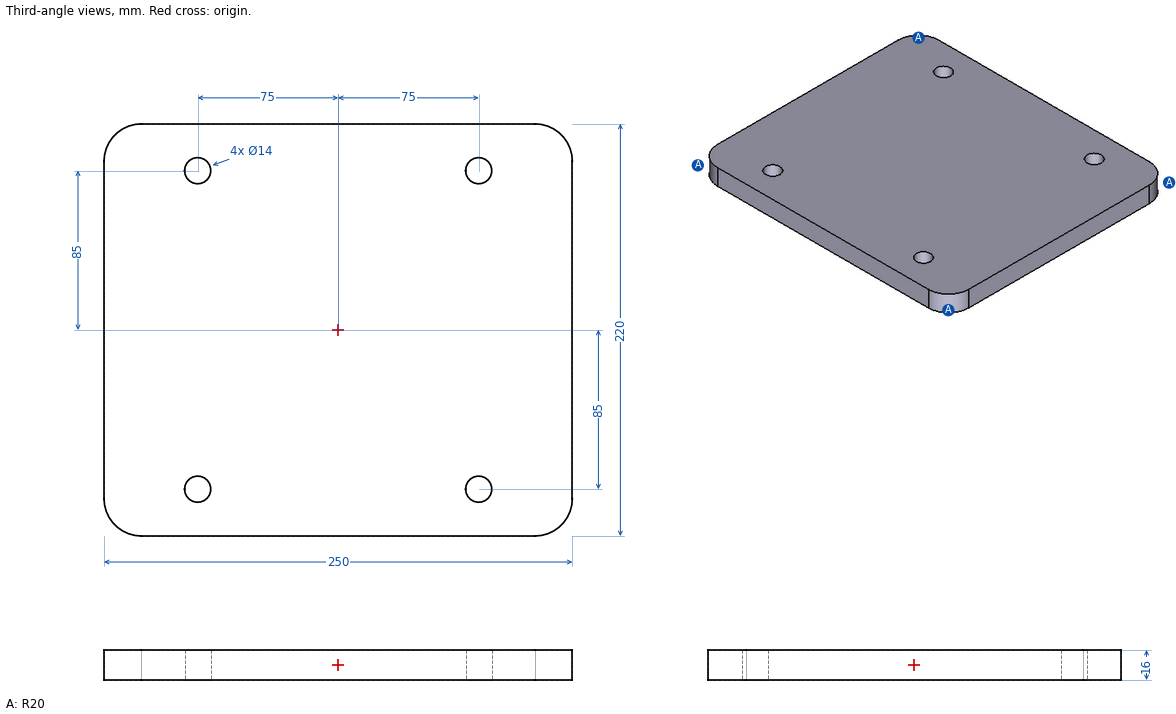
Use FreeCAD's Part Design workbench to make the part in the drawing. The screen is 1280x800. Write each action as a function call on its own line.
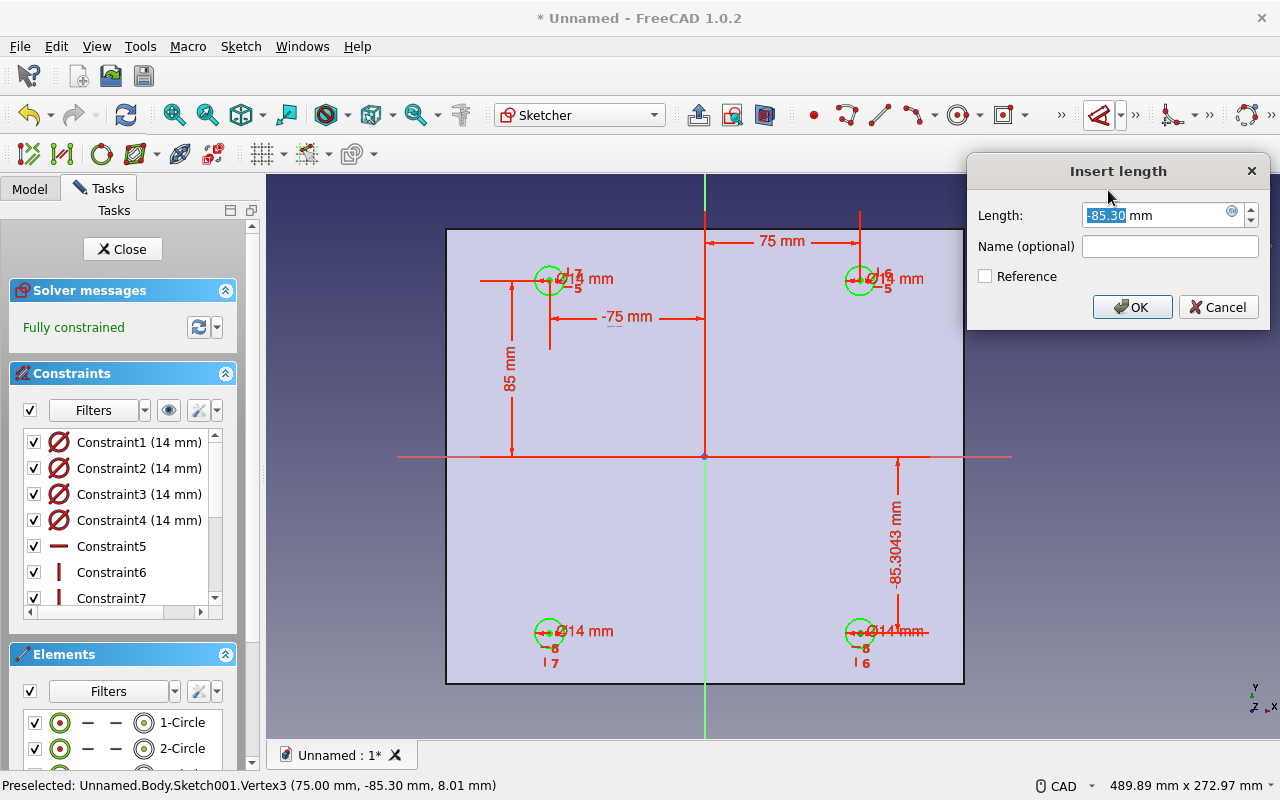
text(-85)
key(Return)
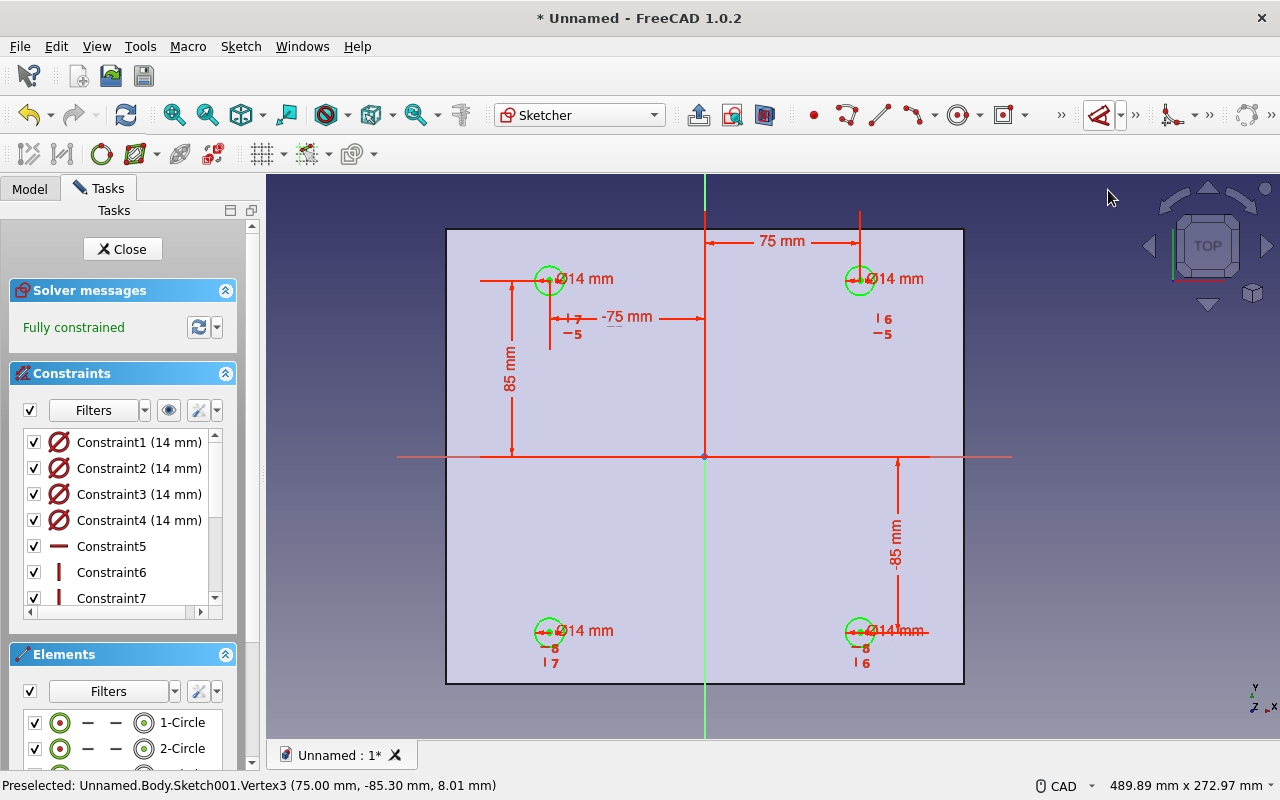
click(123, 249)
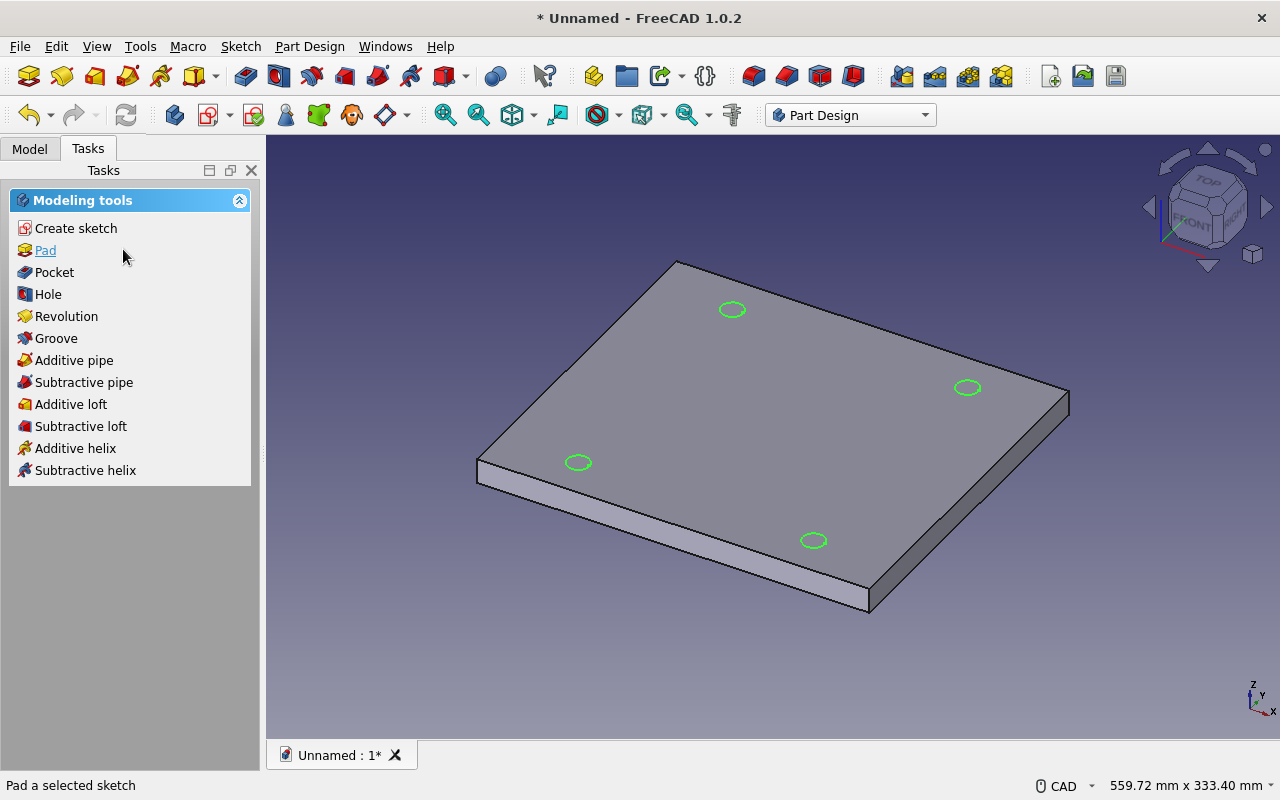
click(246, 76)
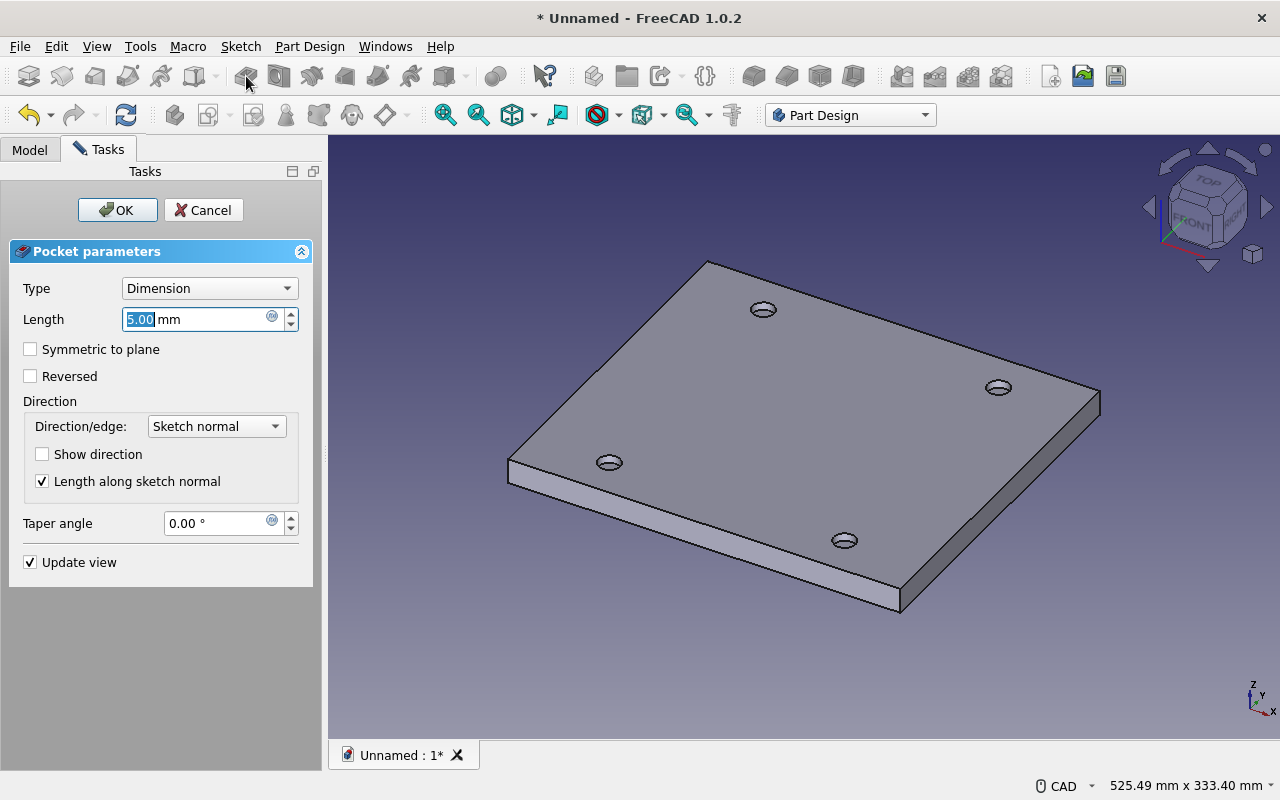
click(210, 288)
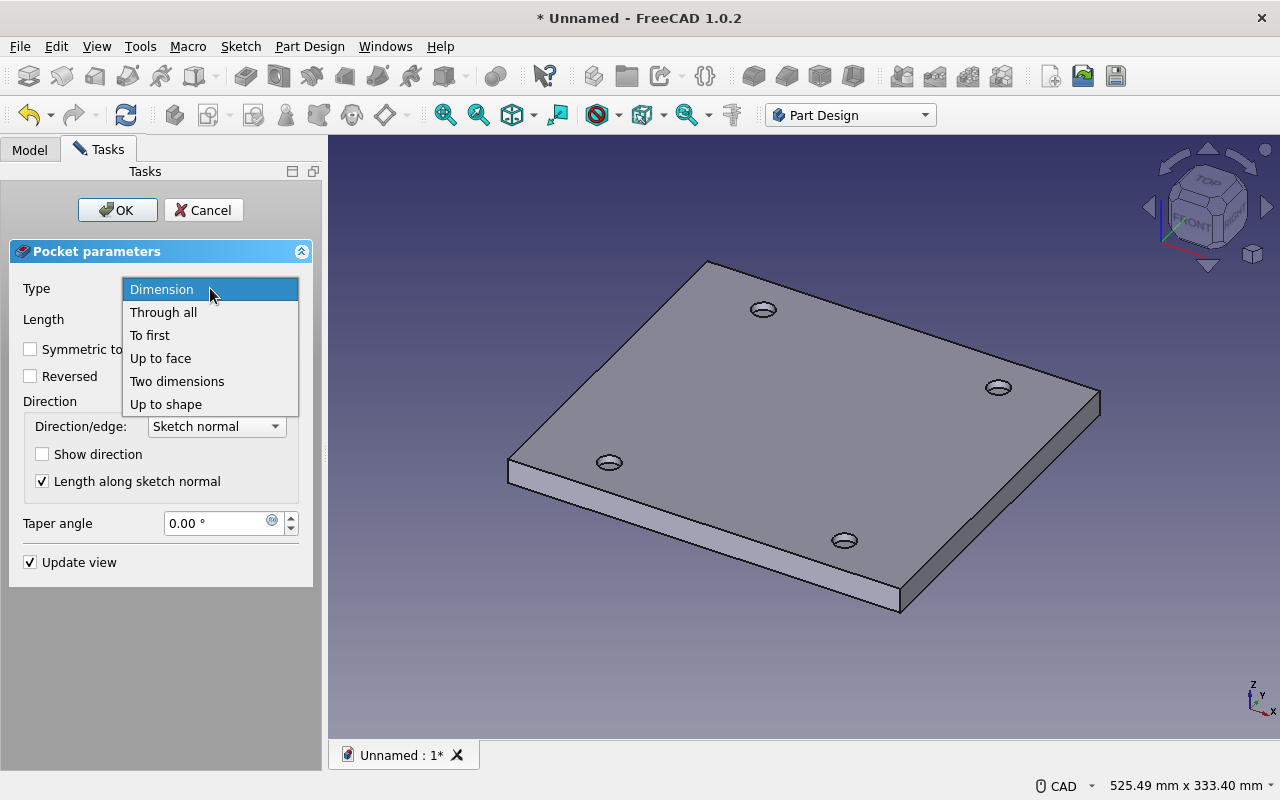
click(208, 312)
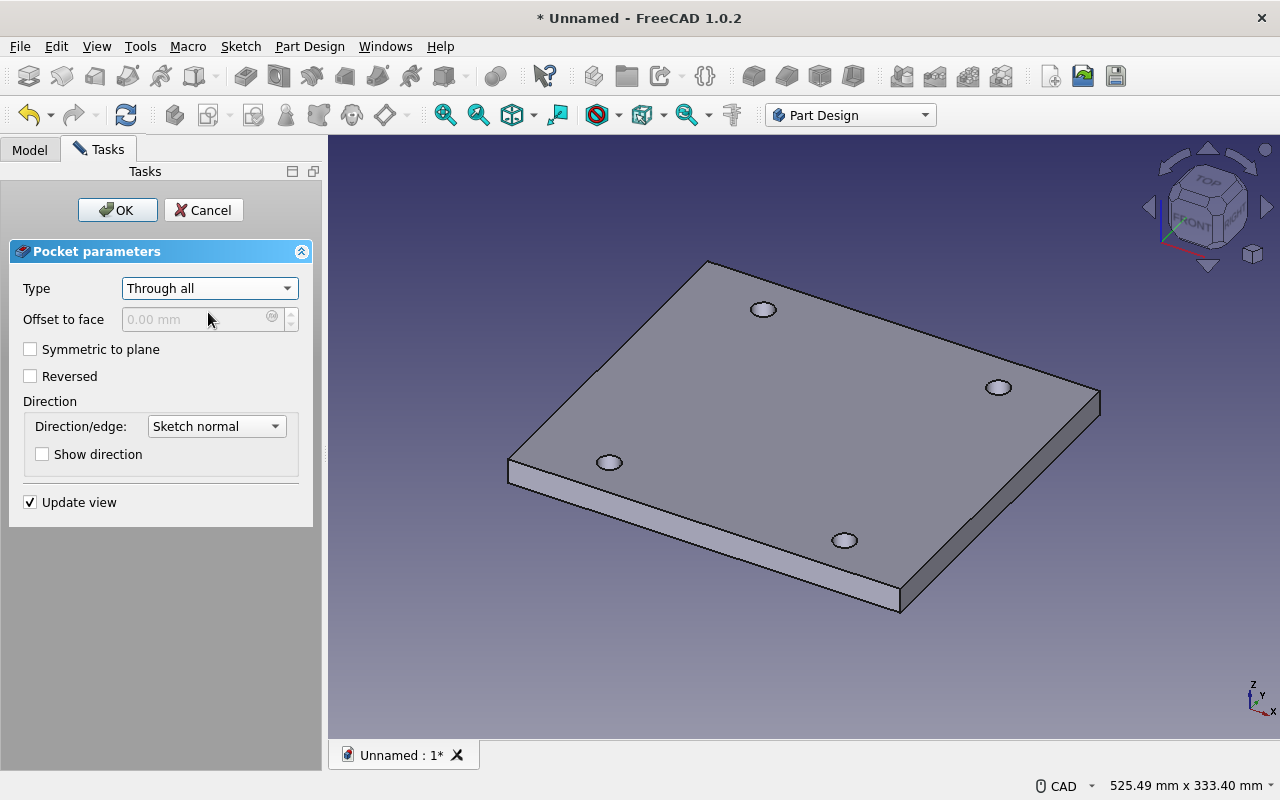
click(118, 210)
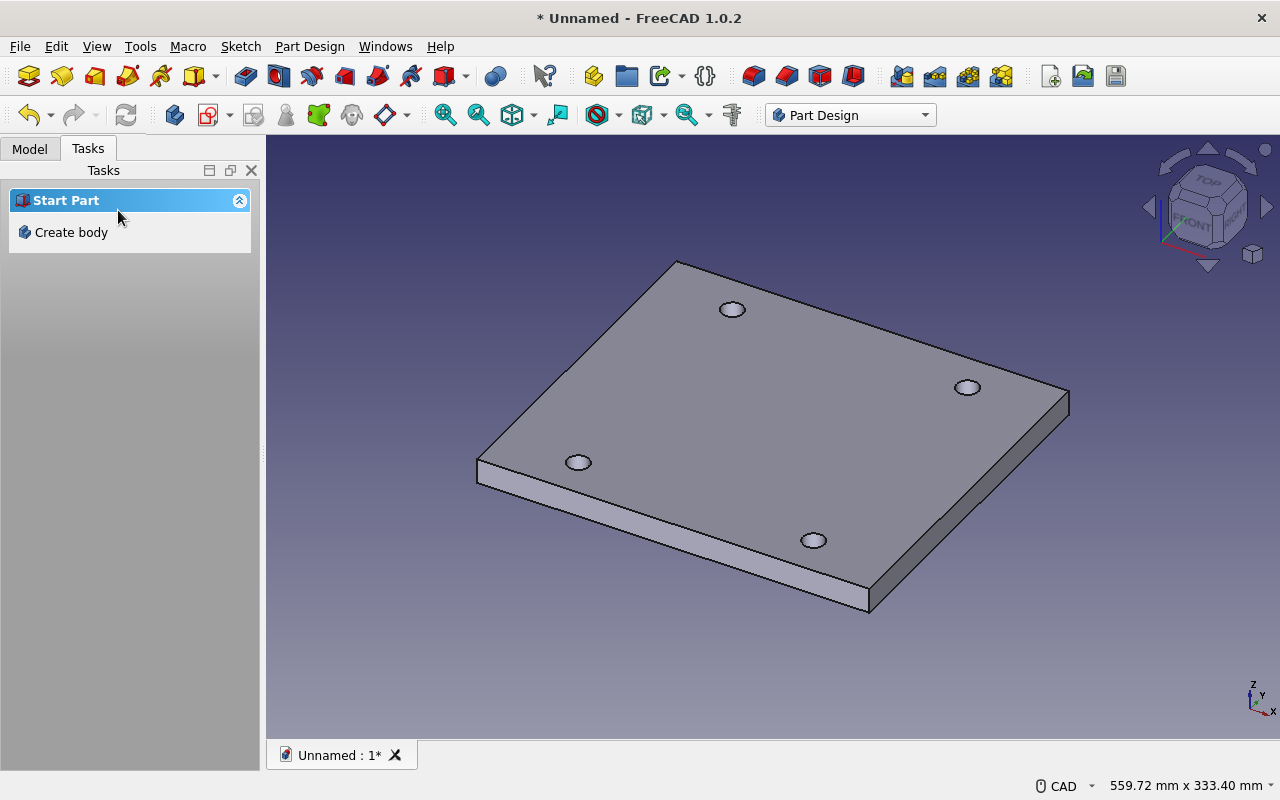
click(869, 600)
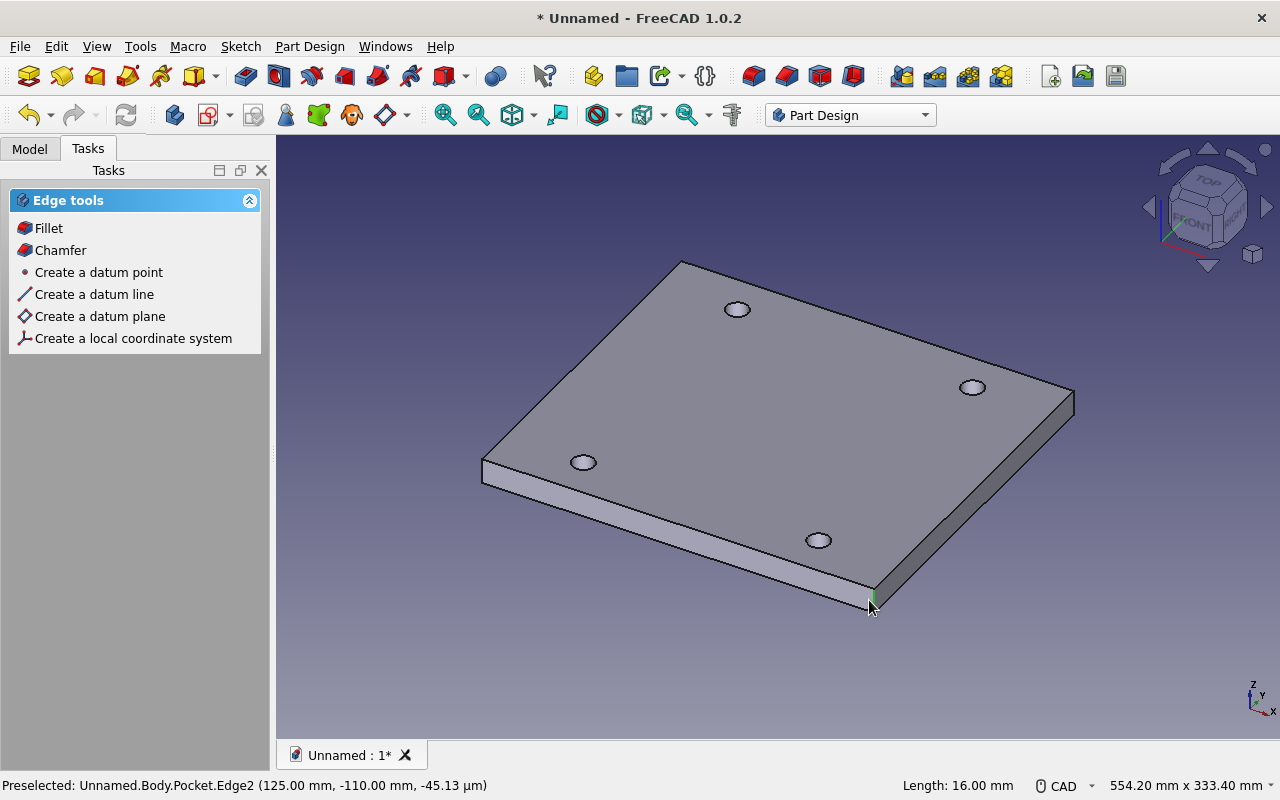
key(0)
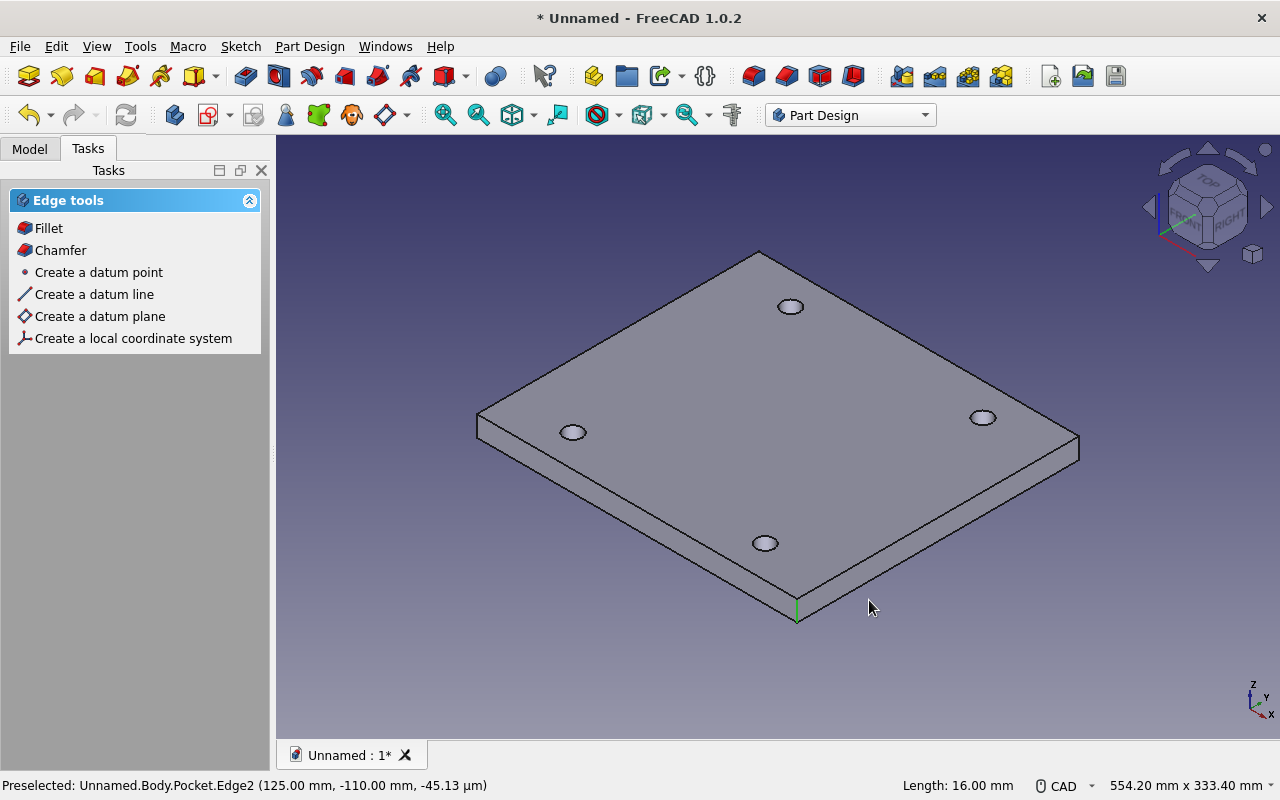
key(2)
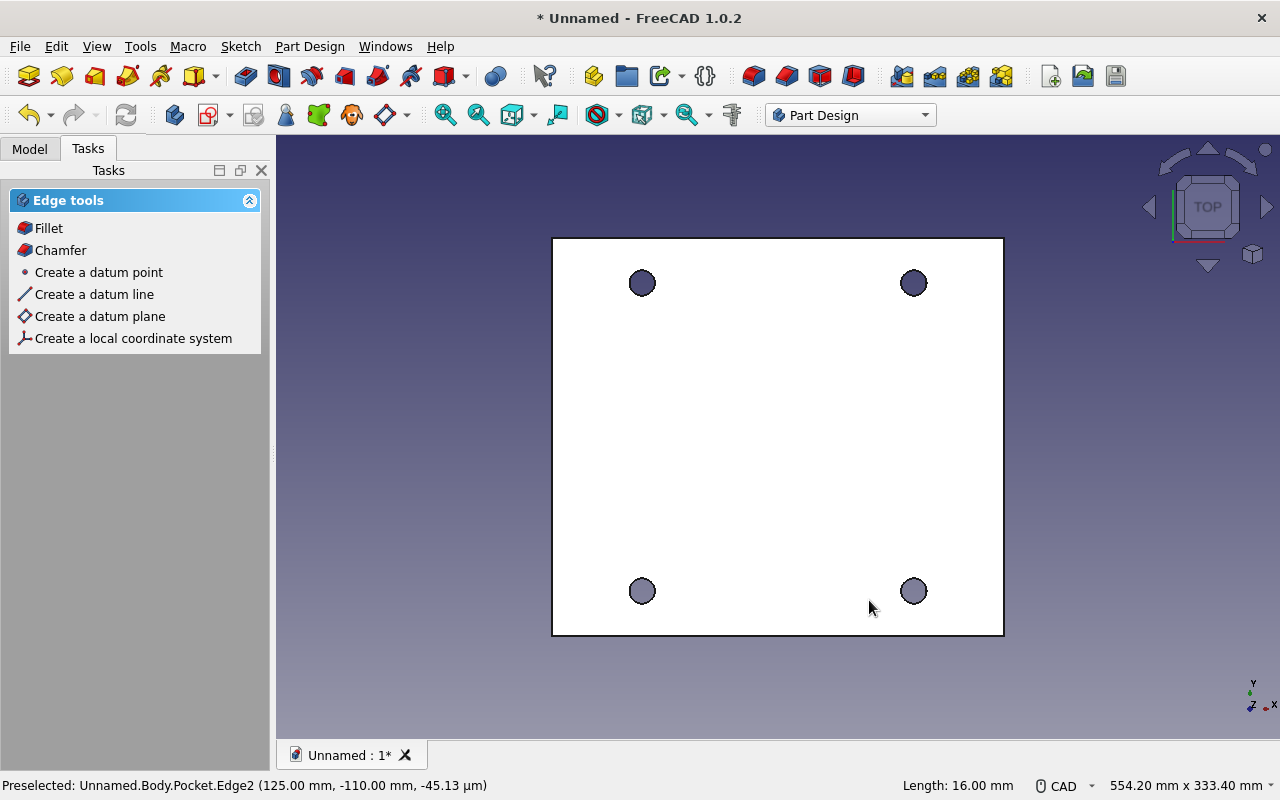
key(1)